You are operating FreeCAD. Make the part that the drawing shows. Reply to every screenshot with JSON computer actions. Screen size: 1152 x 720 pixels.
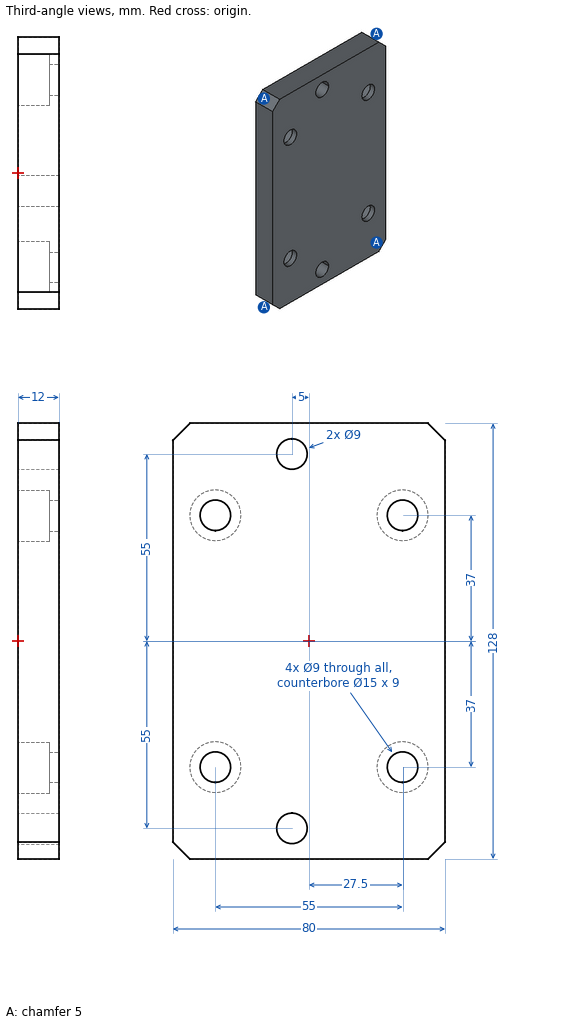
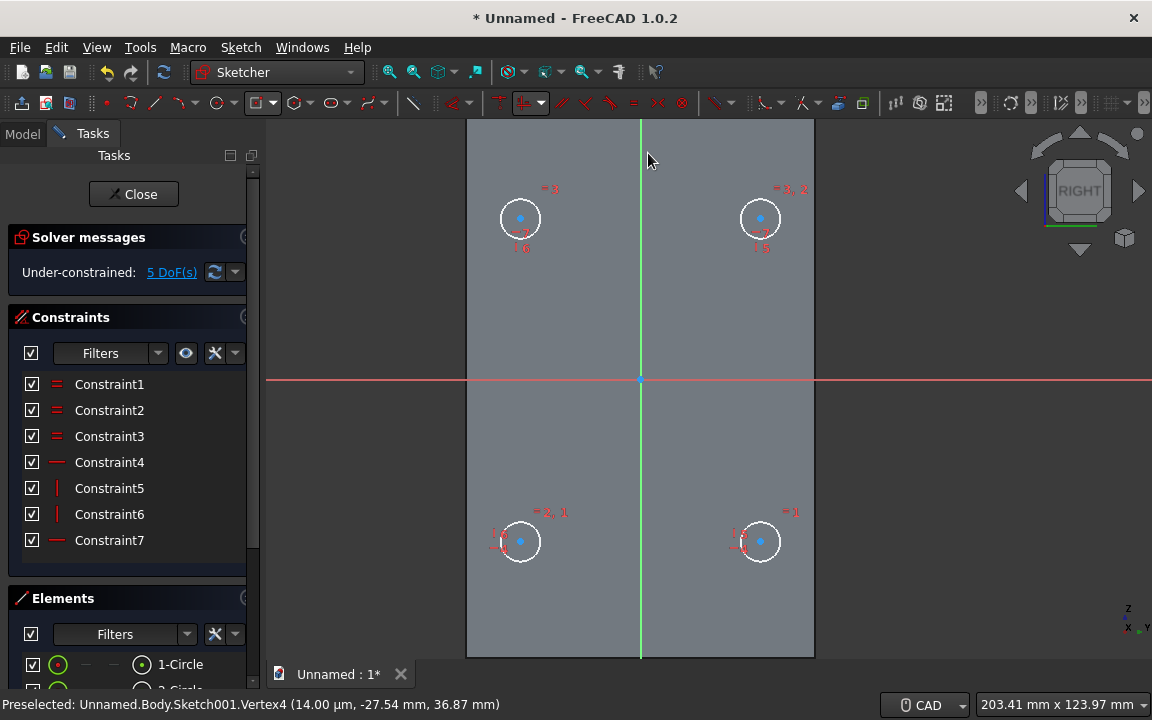
{"action": "left_click", "coordinate": [452, 104]}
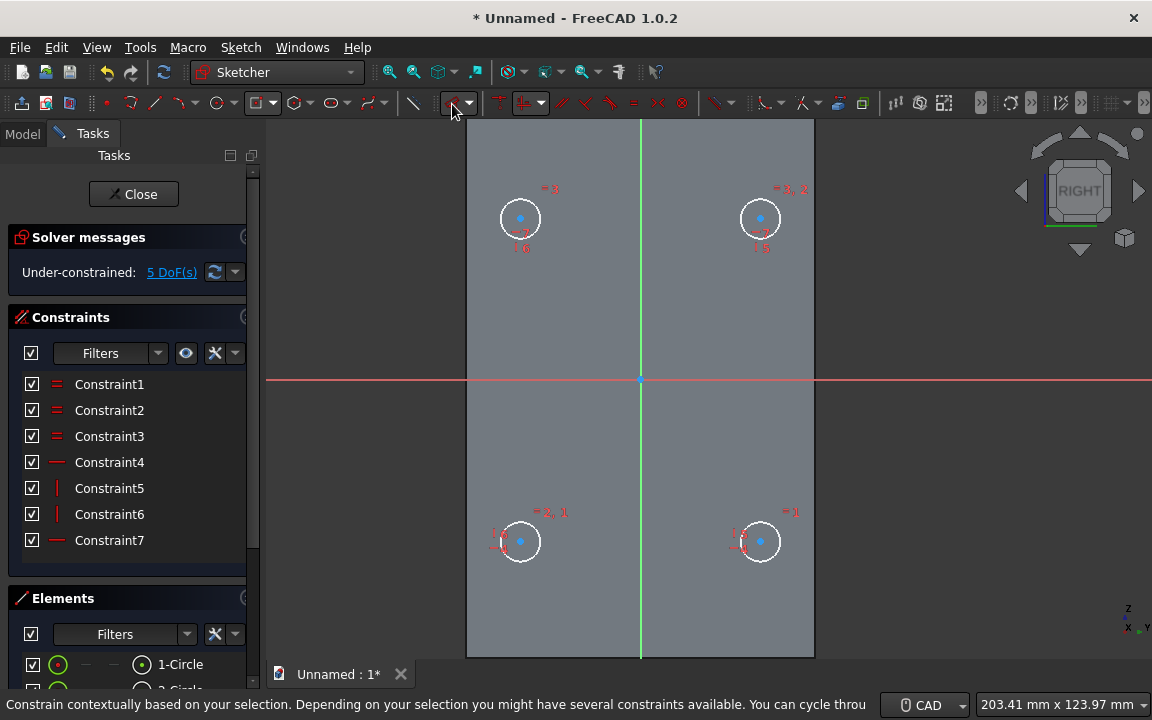
{"action": "left_click", "coordinate": [774, 528]}
{"action": "left_click", "coordinate": [796, 505]}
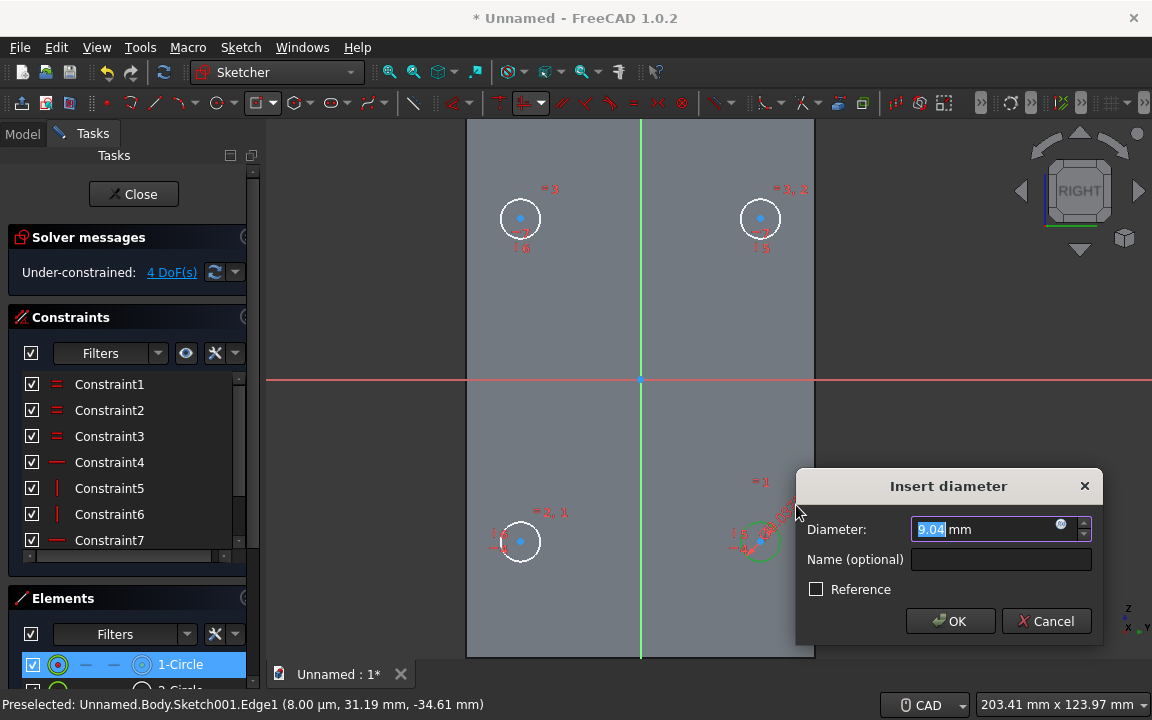
{"action": "type", "text": "9"}
{"action": "key", "text": "Return"}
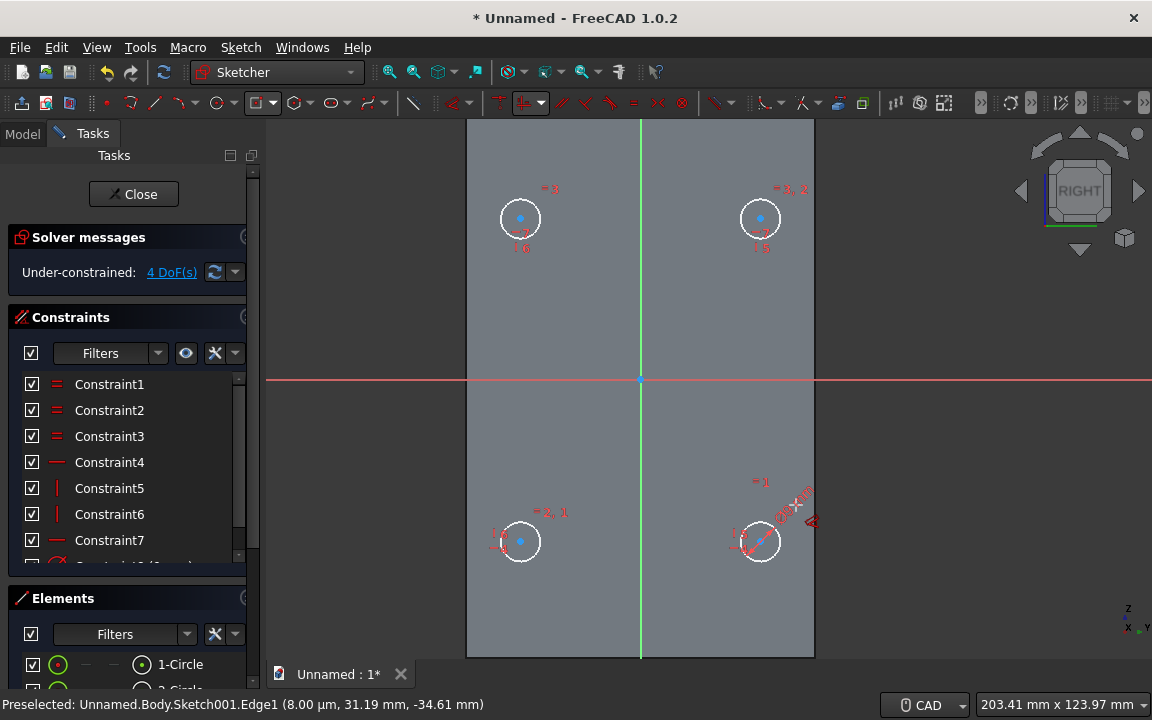
{"action": "left_click", "coordinate": [760, 542]}
{"action": "left_click", "coordinate": [794, 461]}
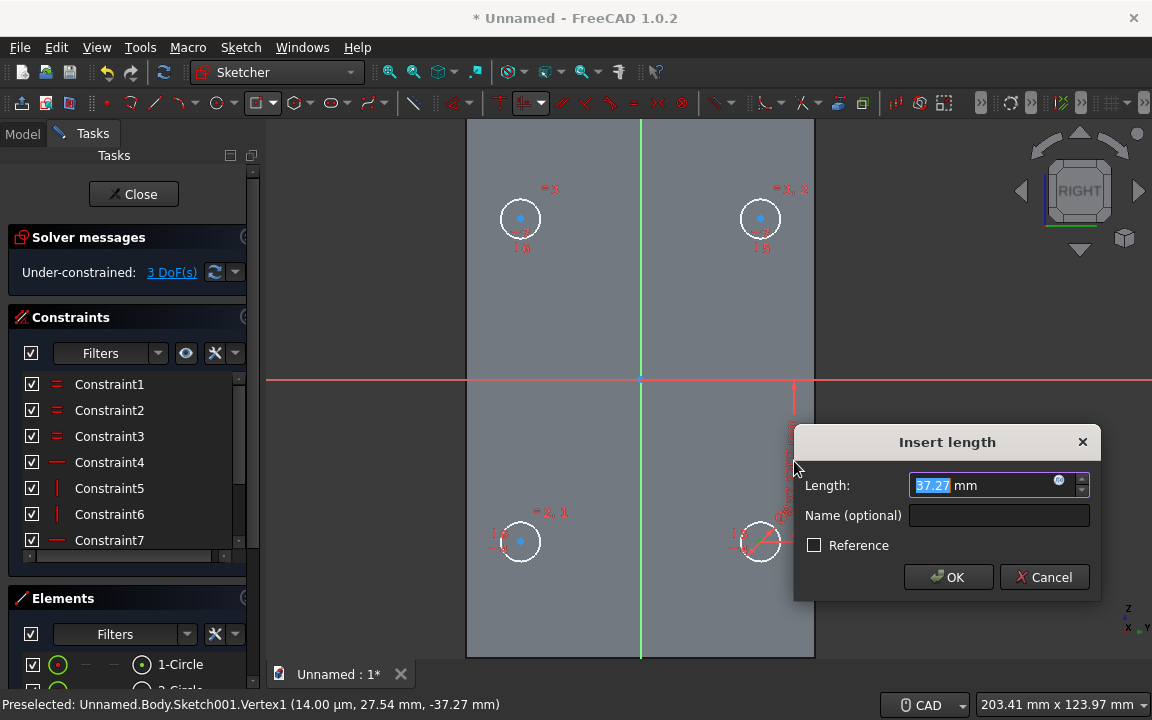
{"action": "type", "text": "37"}
{"action": "key", "text": "Return"}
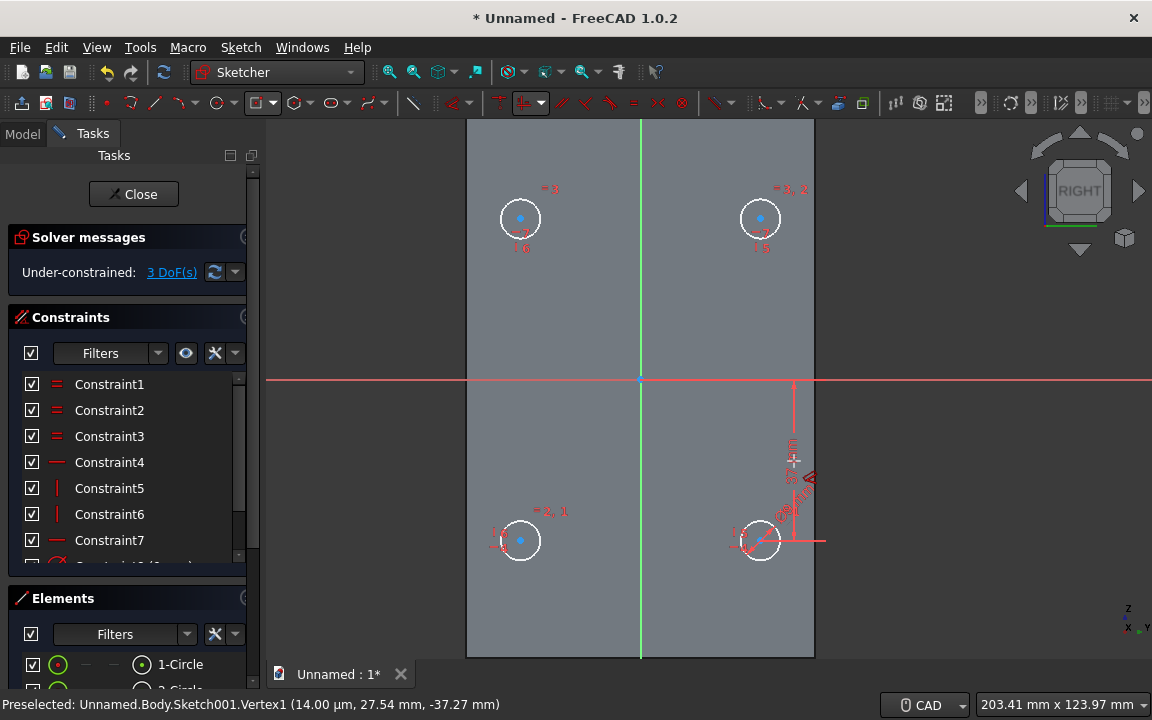
{"action": "left_click", "coordinate": [760, 219]}
{"action": "left_click", "coordinate": [794, 299]}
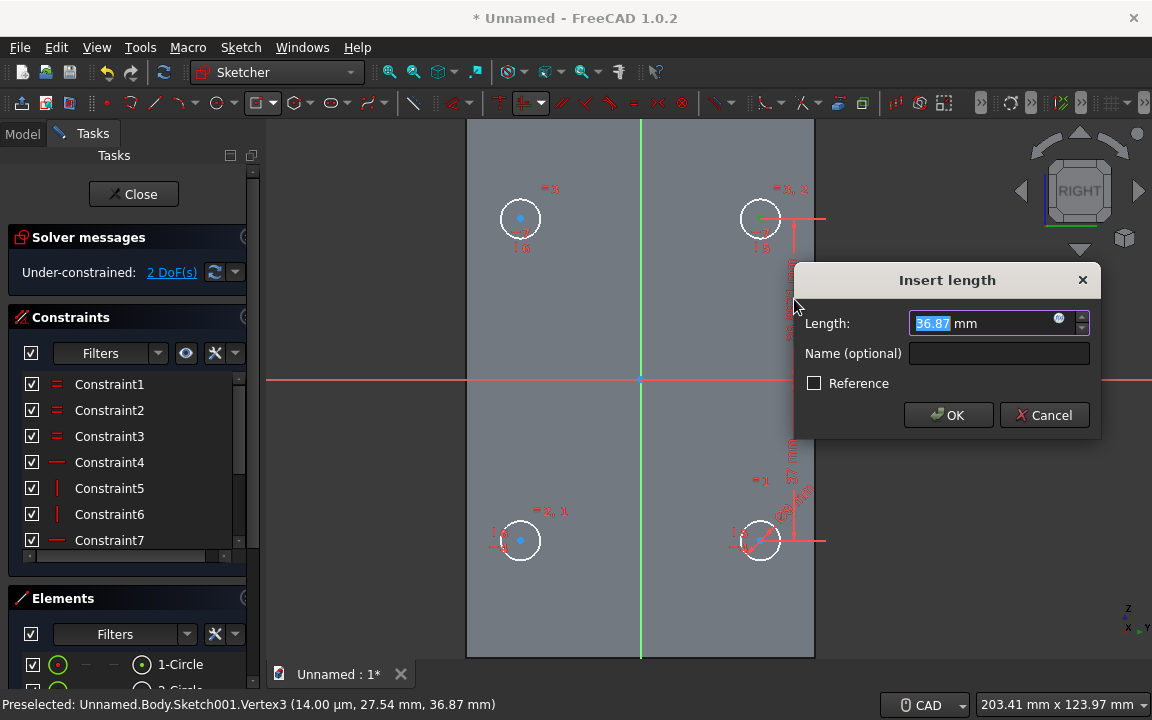
{"action": "type", "text": "37"}
{"action": "key", "text": "Return"}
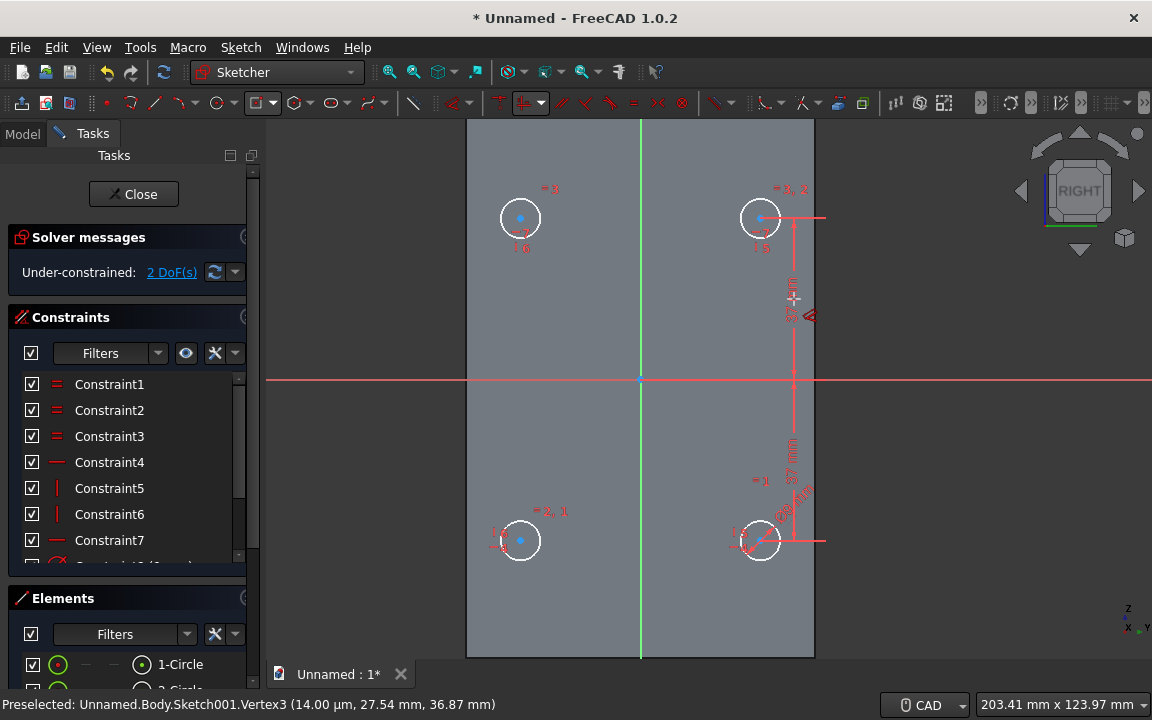
{"action": "left_click", "coordinate": [760, 541]}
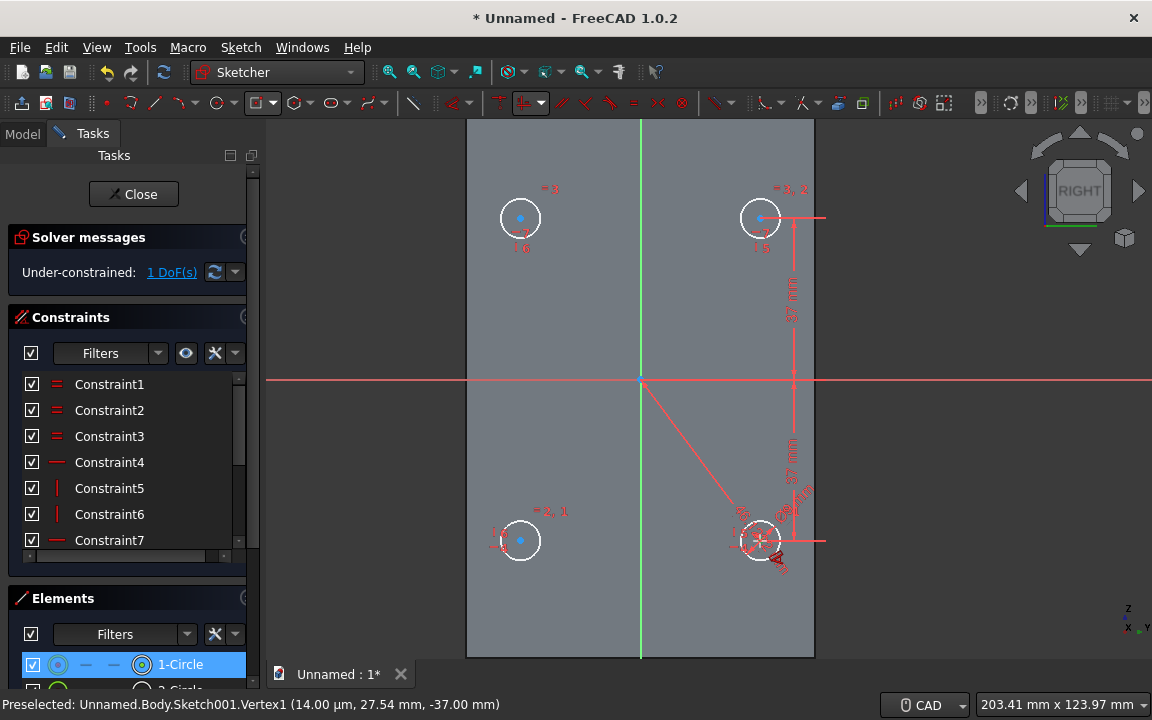
{"action": "left_click", "coordinate": [521, 541]}
{"action": "left_click", "coordinate": [585, 575]}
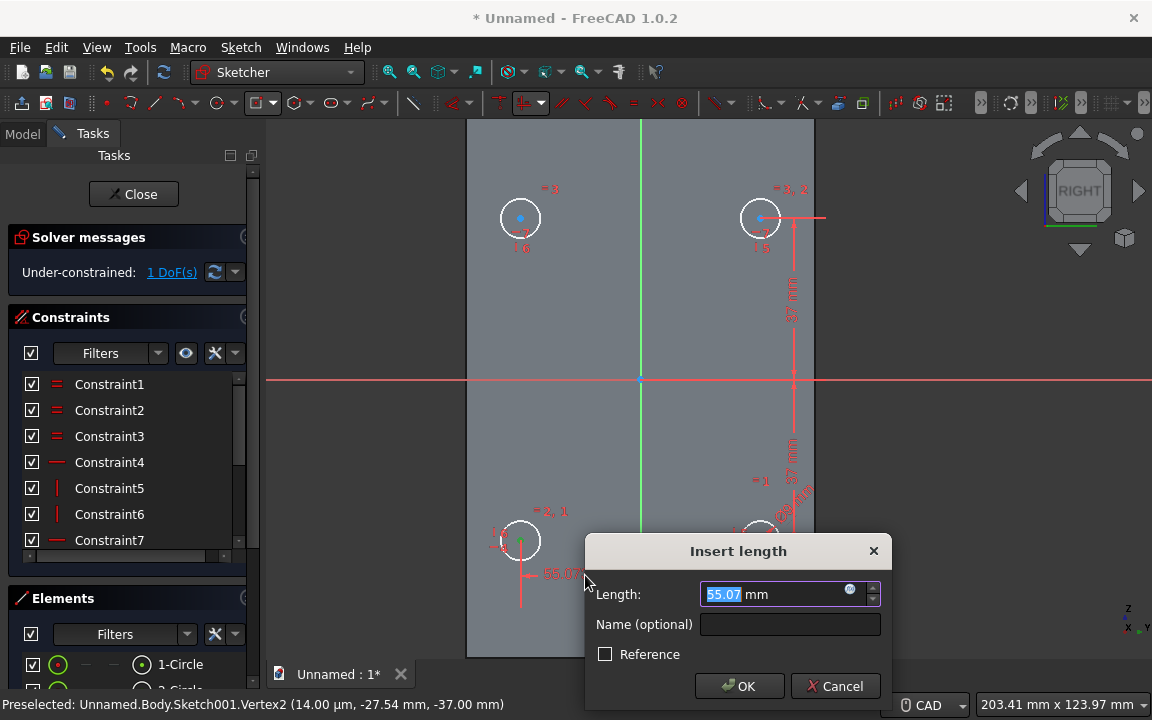
{"action": "type", "text": "55"}
{"action": "key", "text": "Return"}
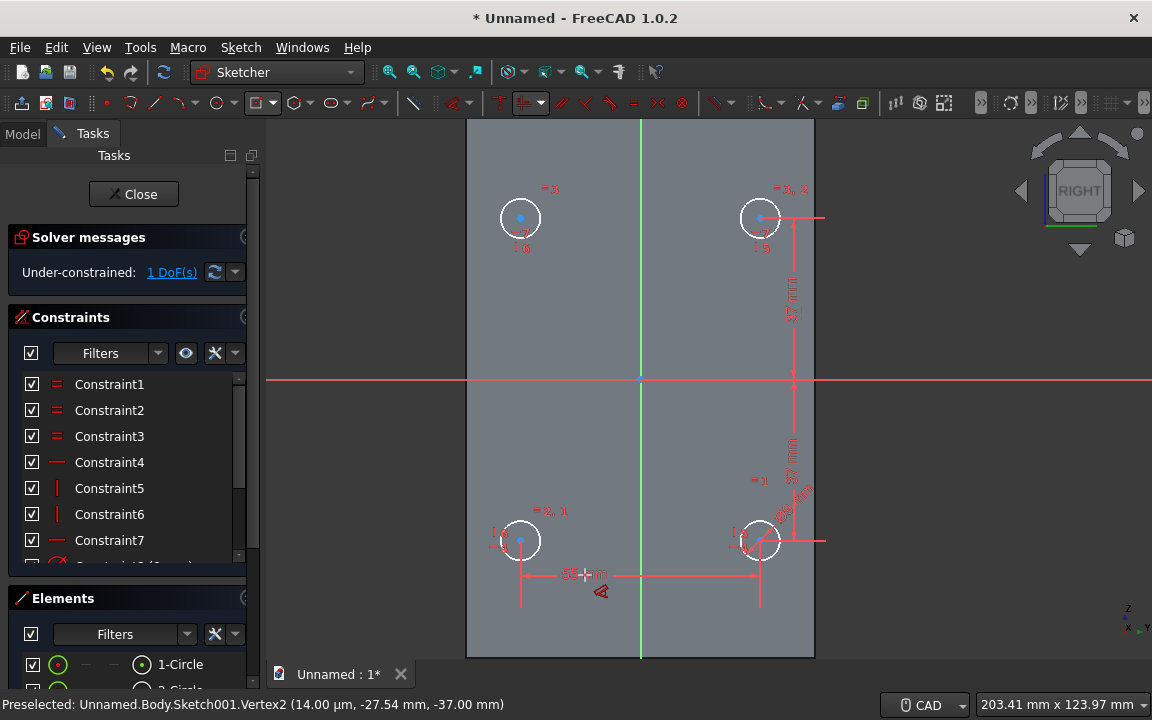
{"action": "left_click", "coordinate": [760, 541]}
{"action": "left_click", "coordinate": [700, 575]}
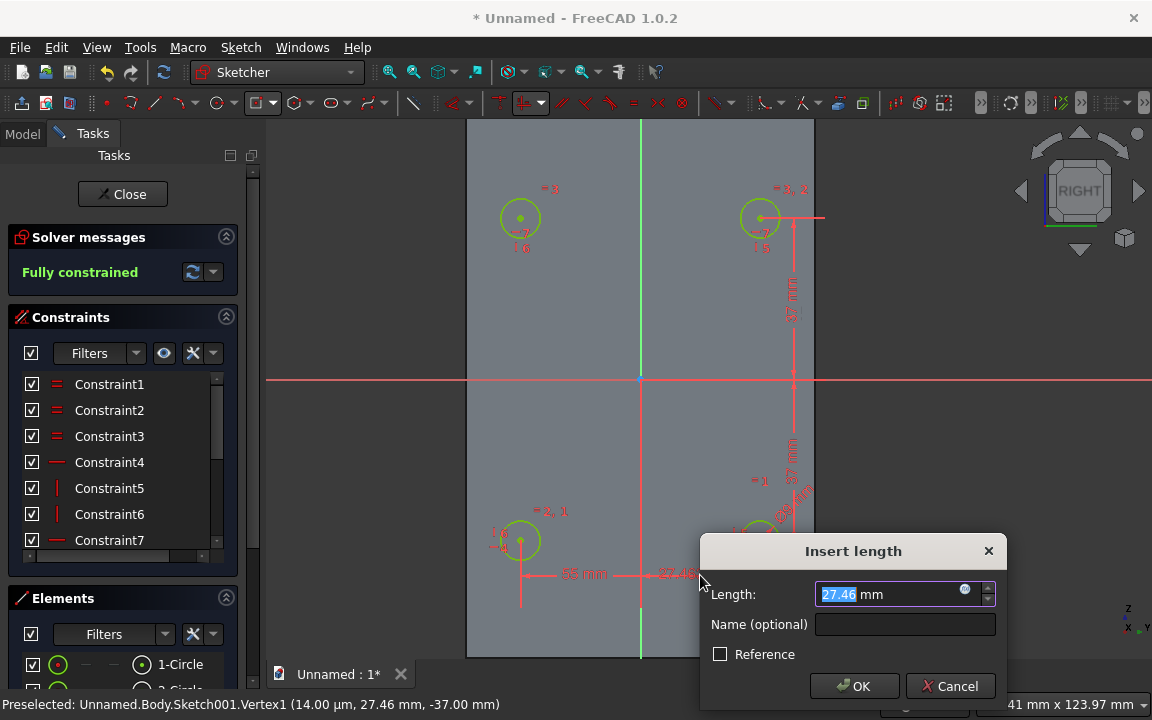
{"action": "type", "text": "27.5"}
{"action": "key", "text": "Return"}
{"action": "key", "text": "Escape"}